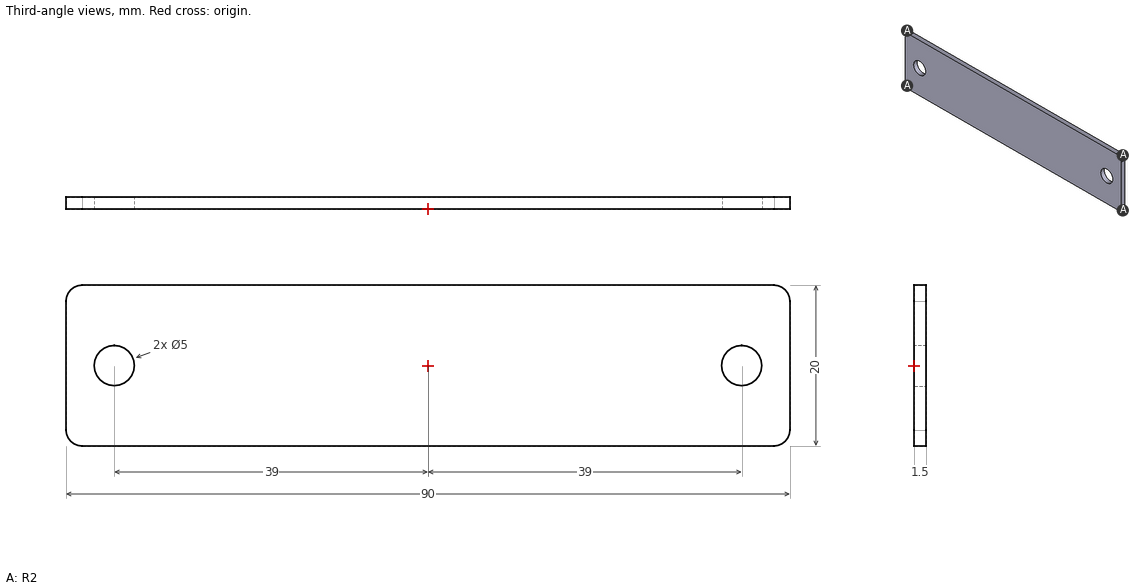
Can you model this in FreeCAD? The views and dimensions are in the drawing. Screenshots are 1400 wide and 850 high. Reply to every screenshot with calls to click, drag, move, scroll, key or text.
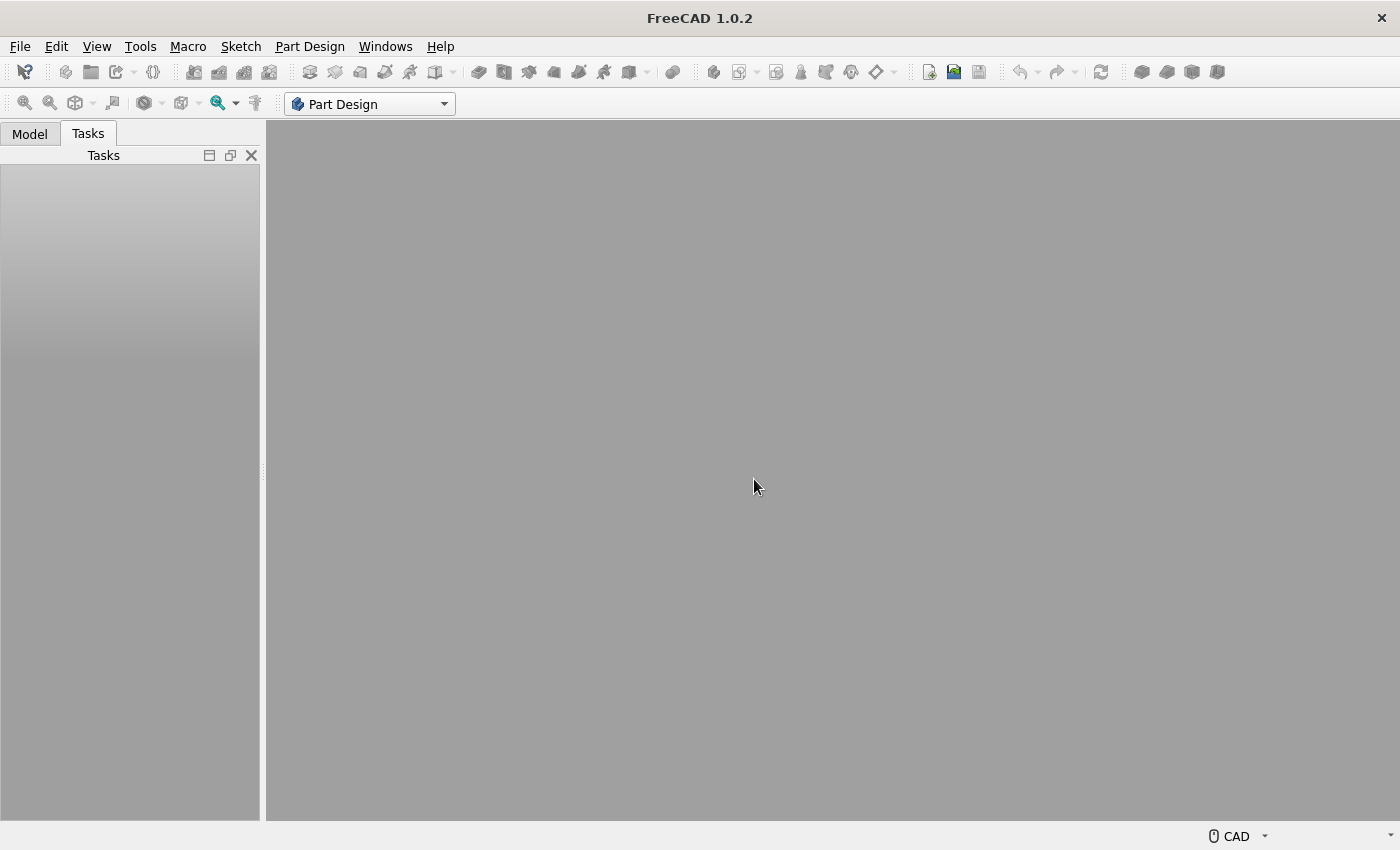
click(929, 72)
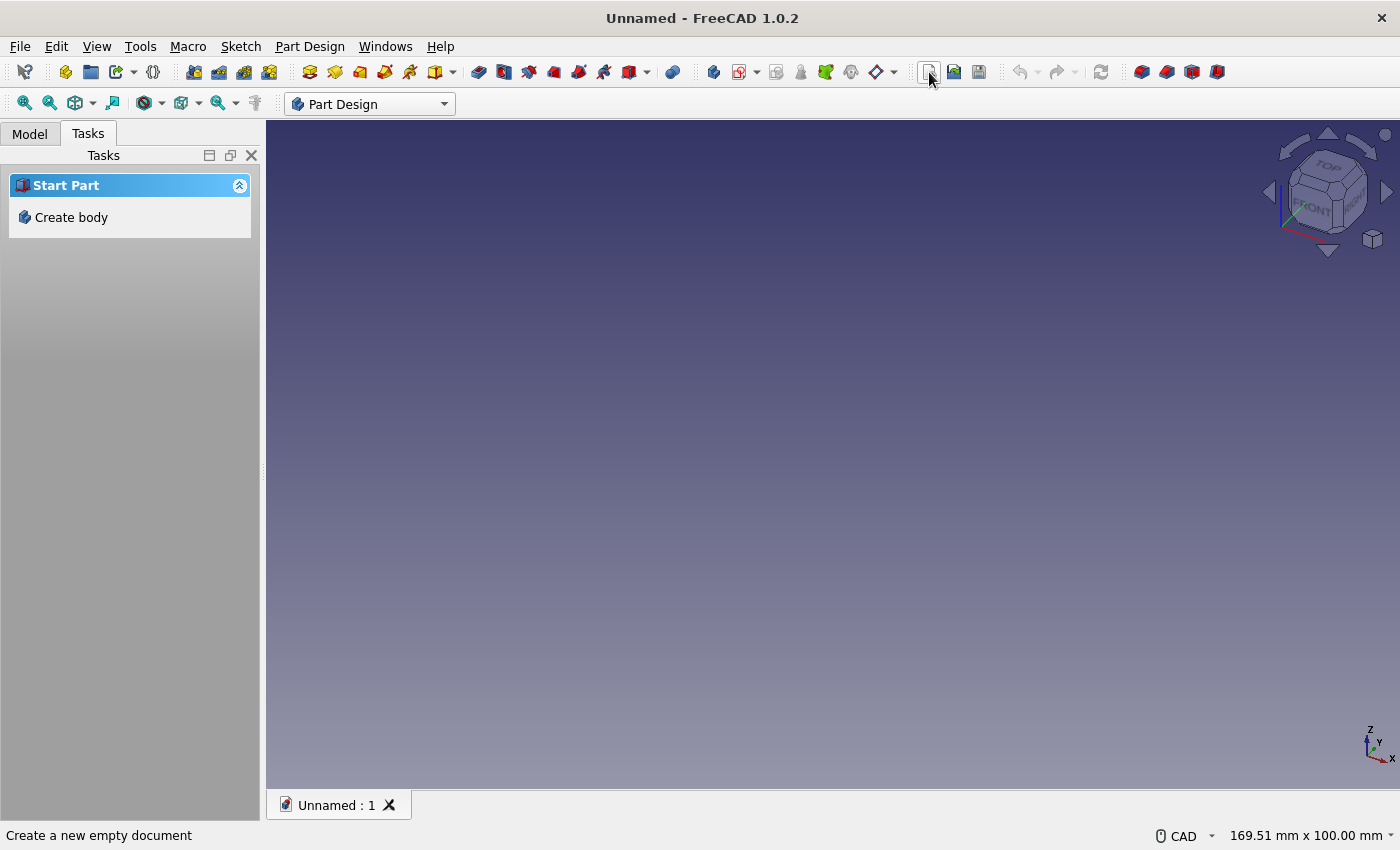
click(738, 72)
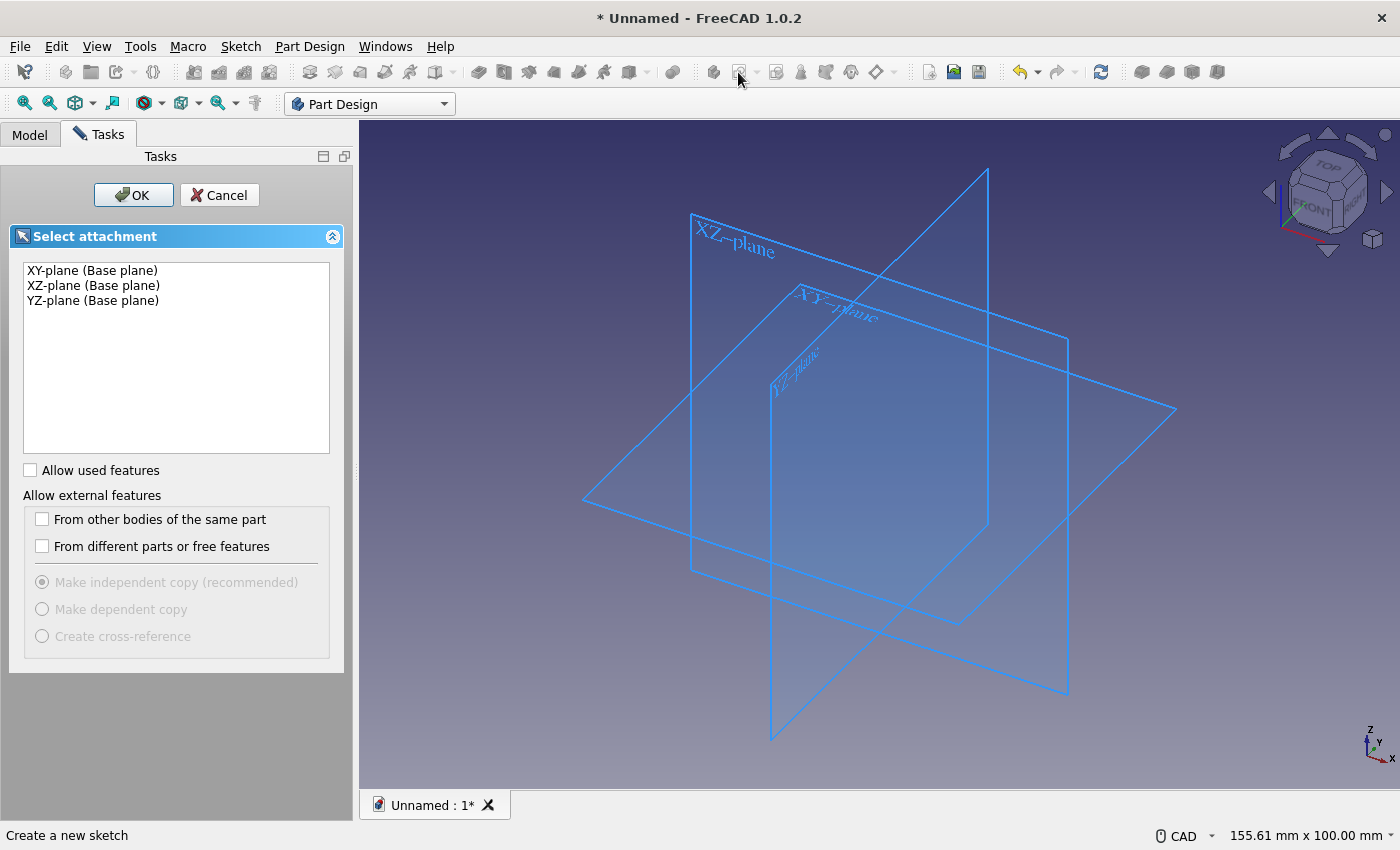
click(84, 286)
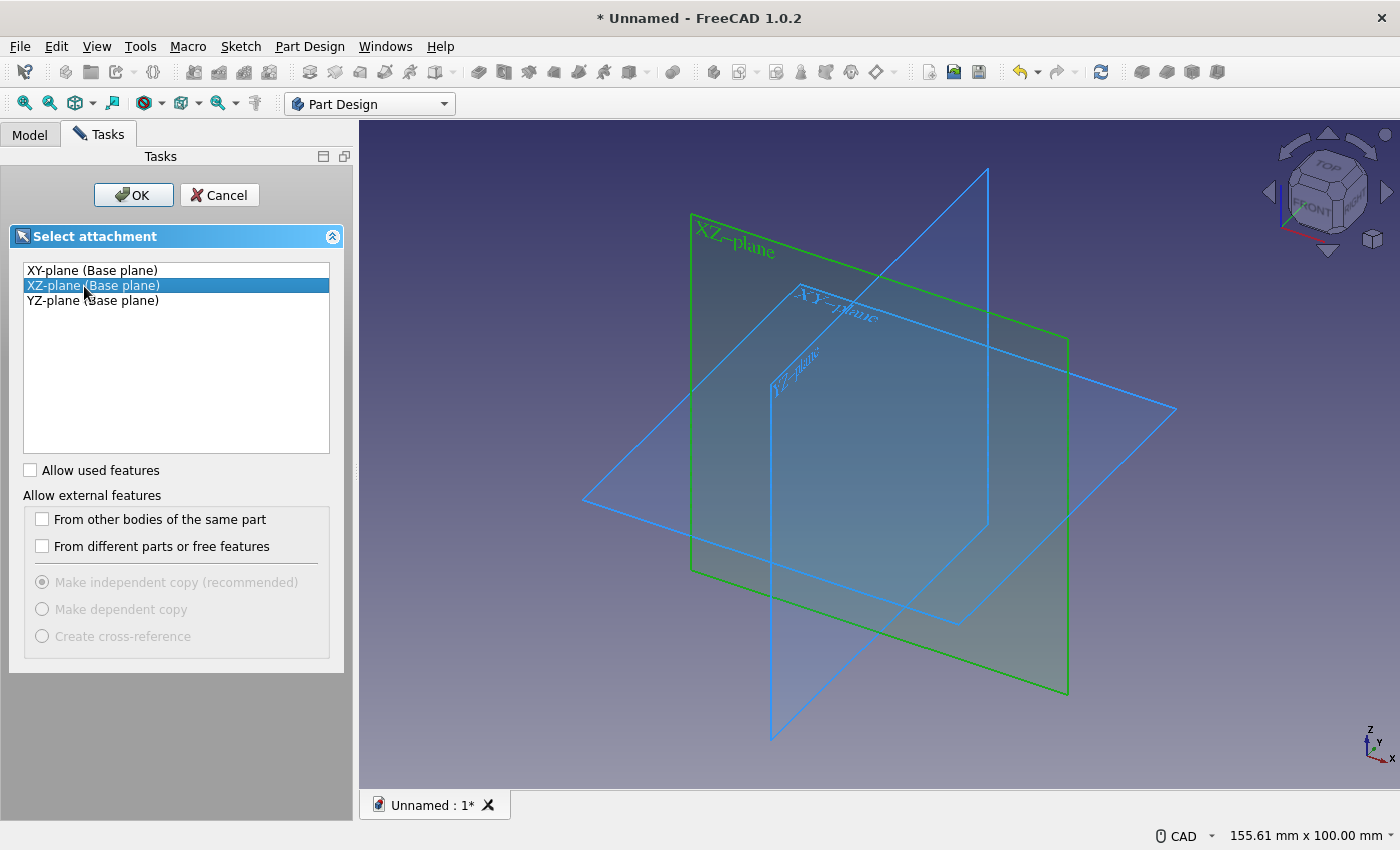
click(134, 195)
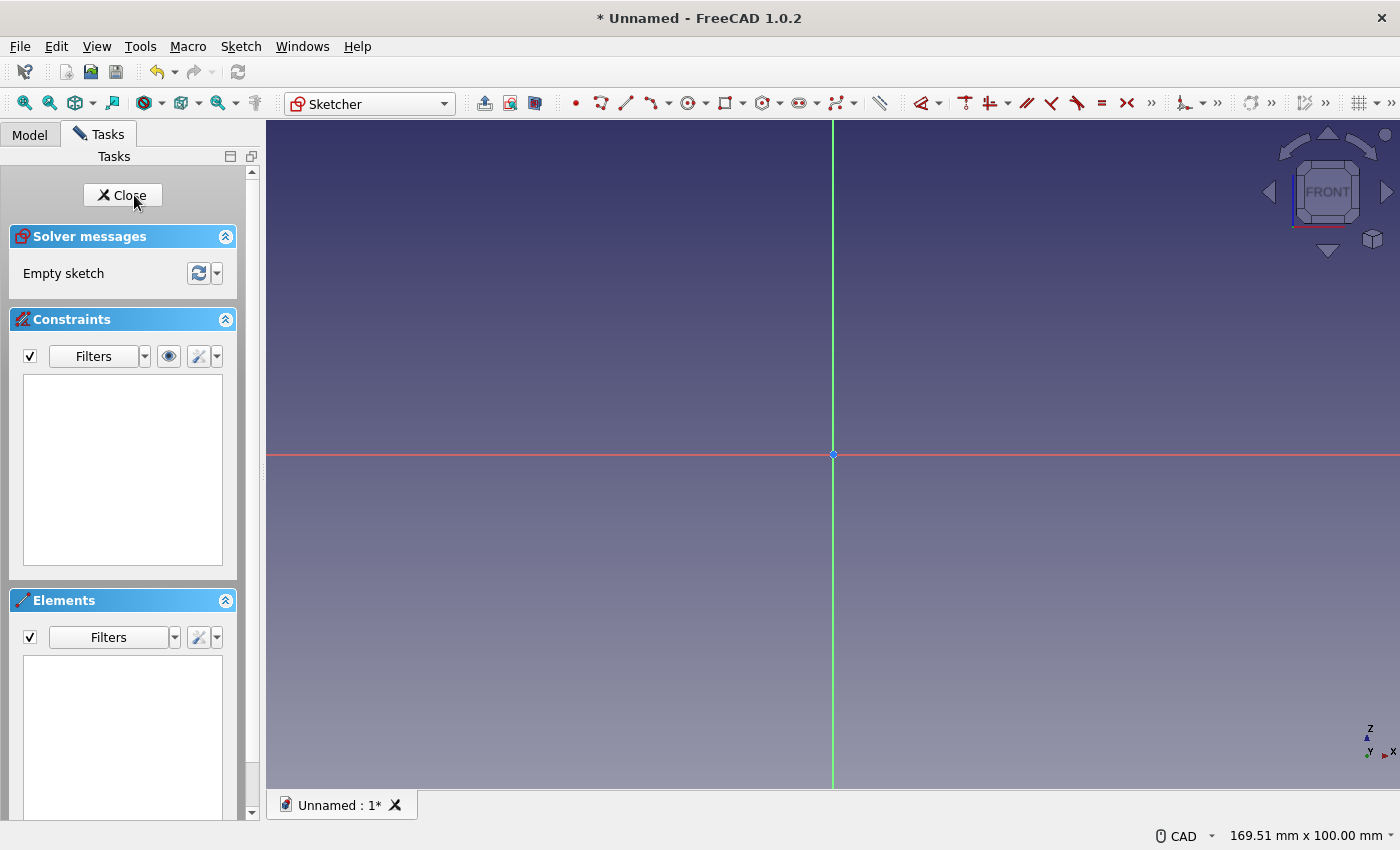
click(742, 104)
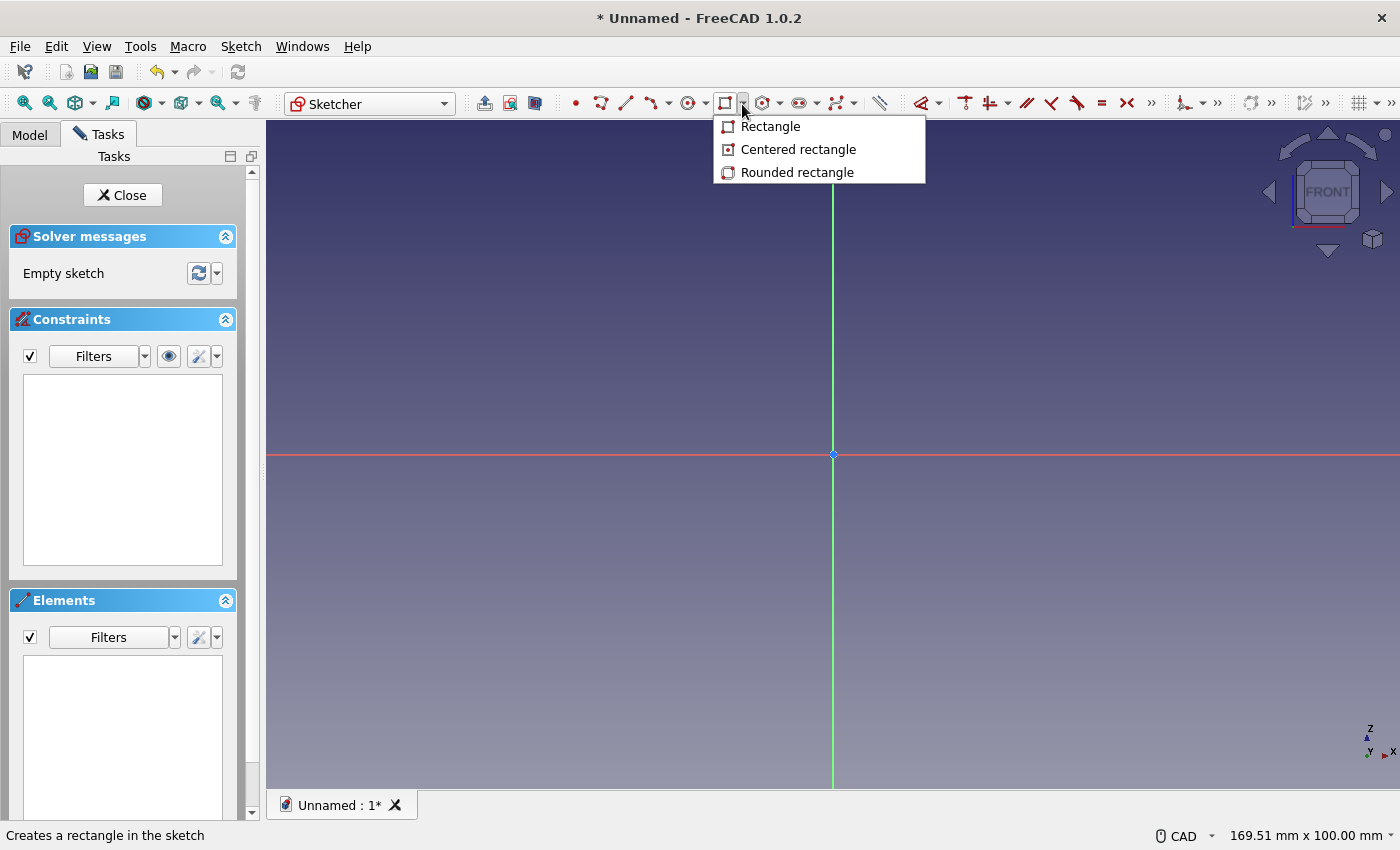
click(820, 150)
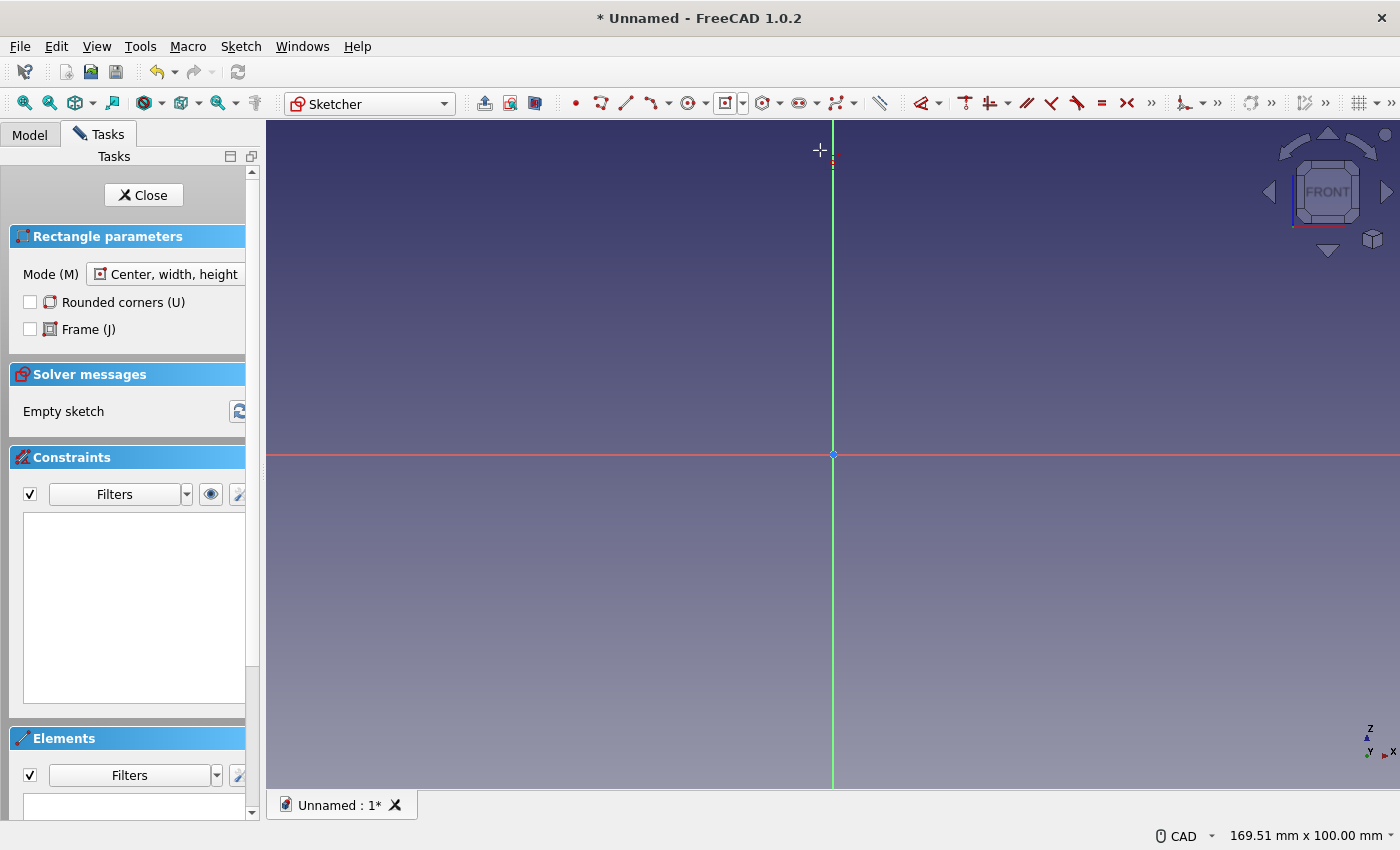
click(833, 454)
move(1134, 388)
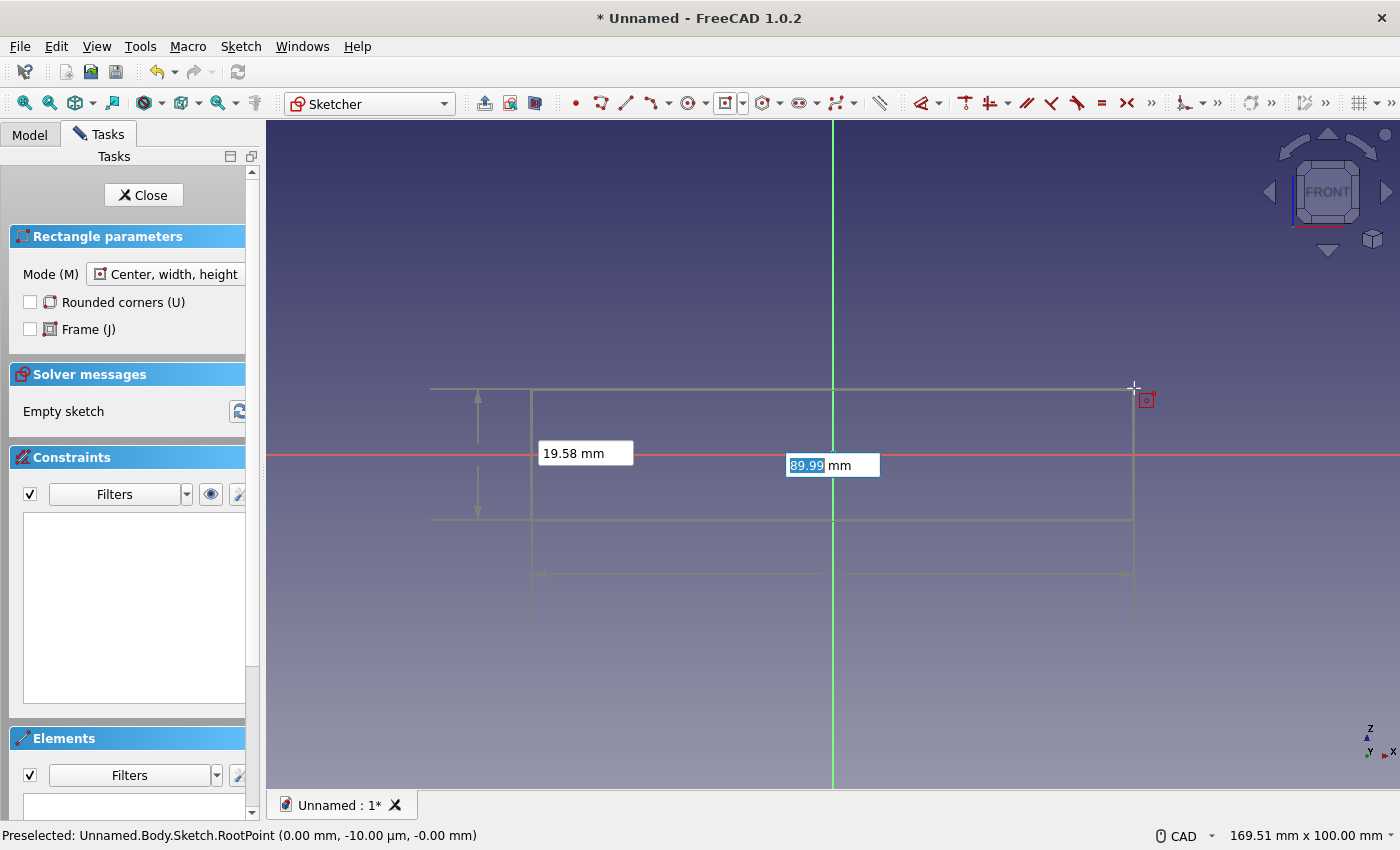
text(90)
key(Tab)
text(20)
key(Return)
key(Escape)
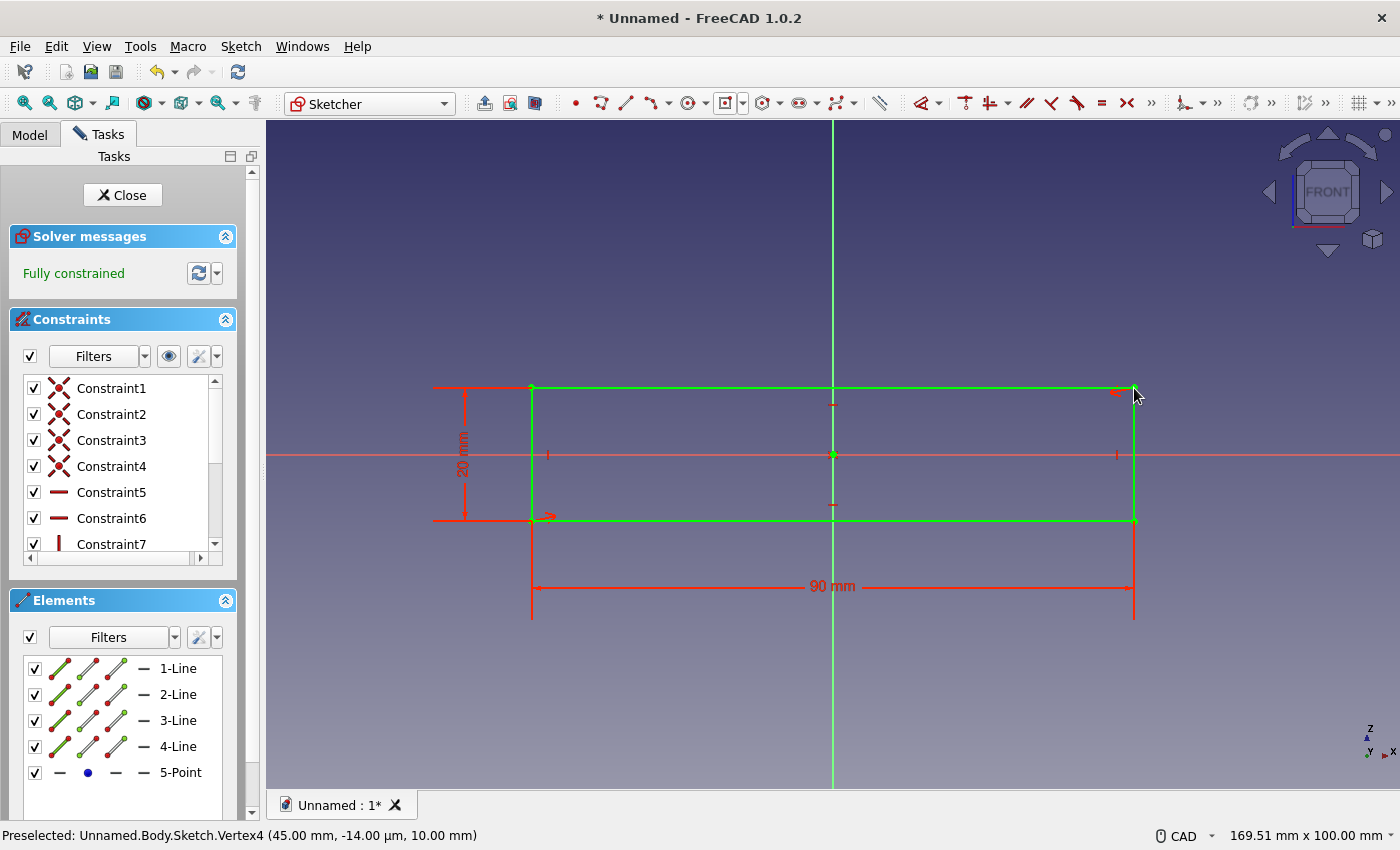
click(123, 195)